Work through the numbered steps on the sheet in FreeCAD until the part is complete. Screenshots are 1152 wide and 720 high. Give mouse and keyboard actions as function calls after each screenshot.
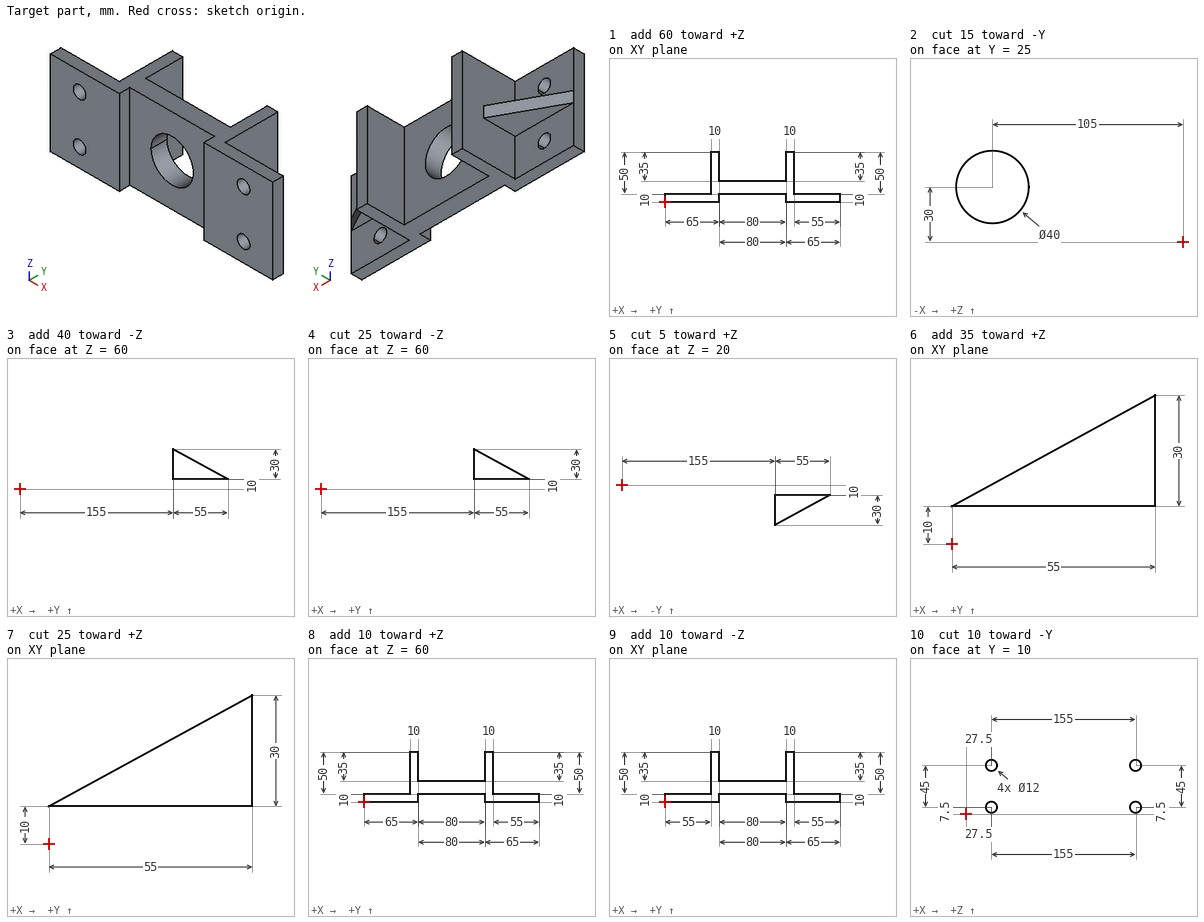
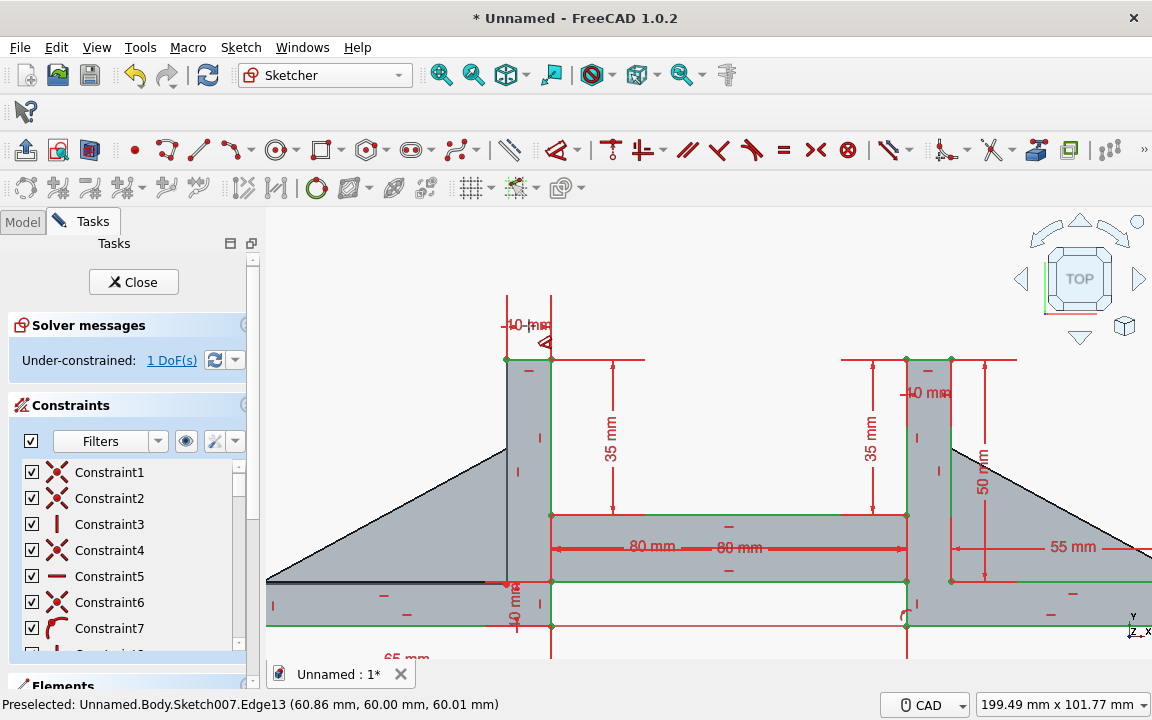
click(507, 427)
click(473, 472)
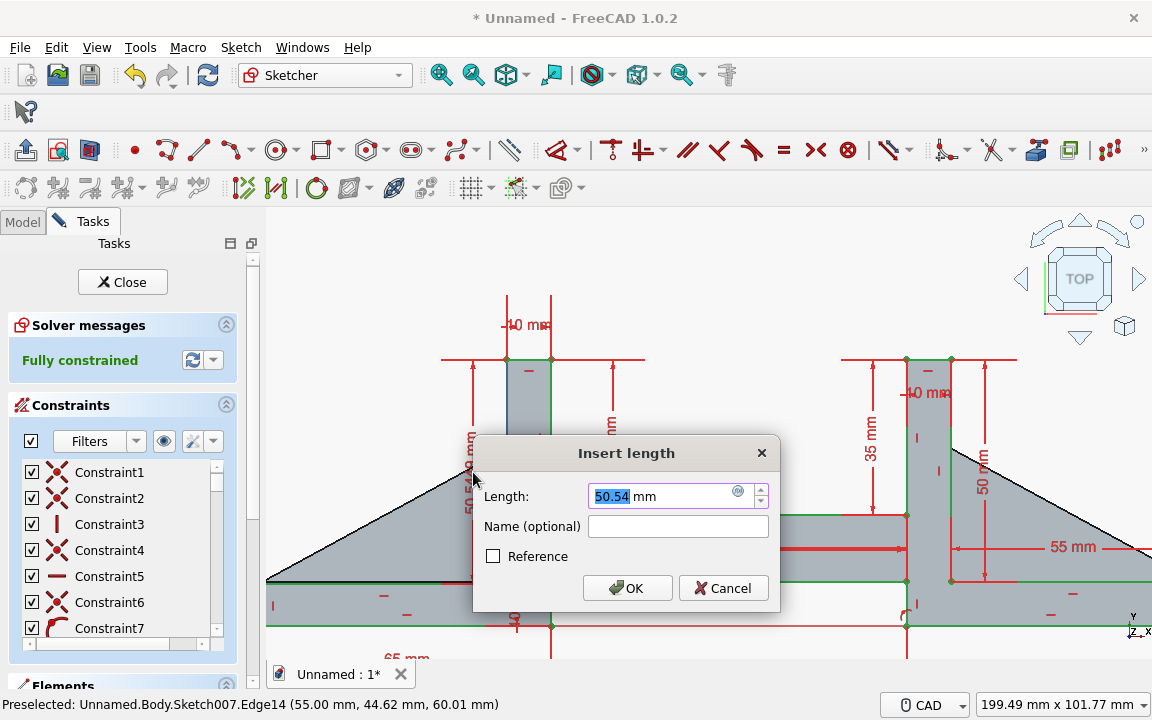
text(50)
key(Return)
key(Escape)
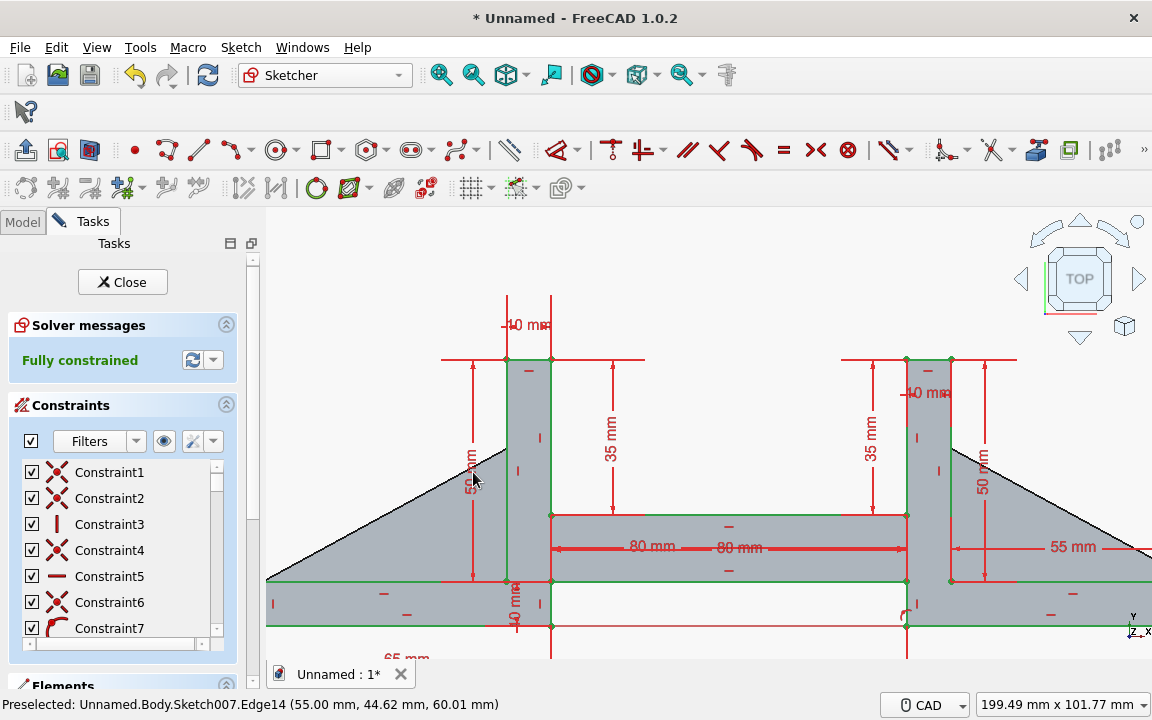
click(123, 282)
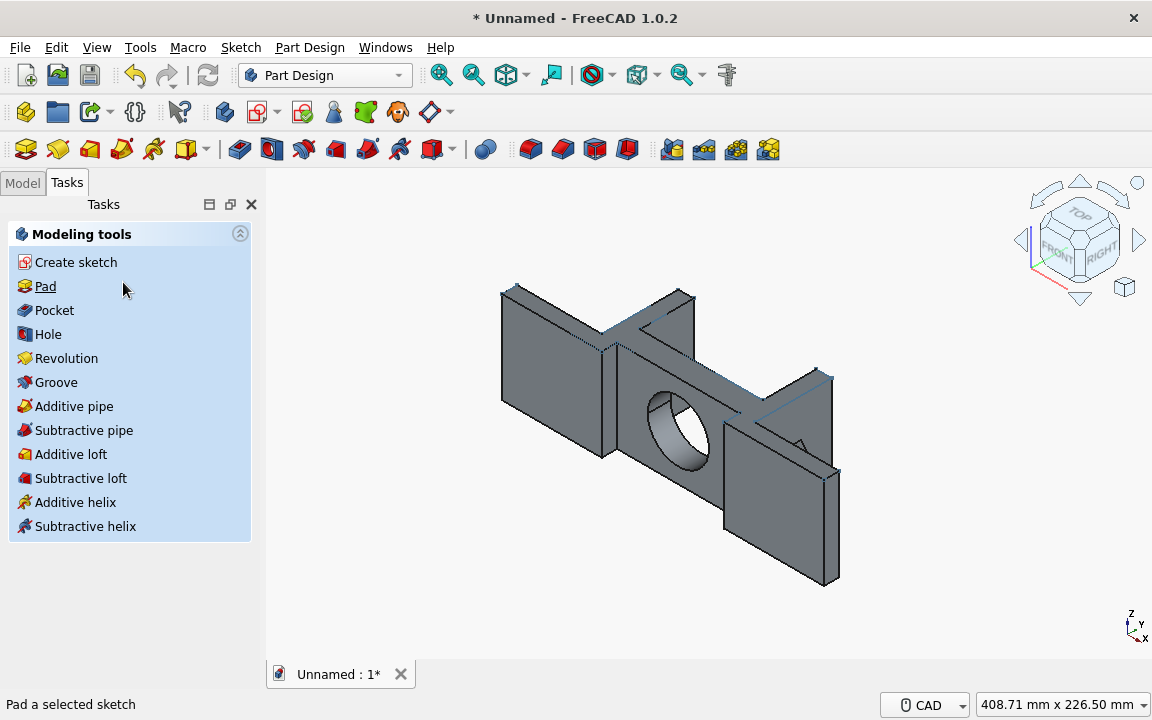
click(26, 150)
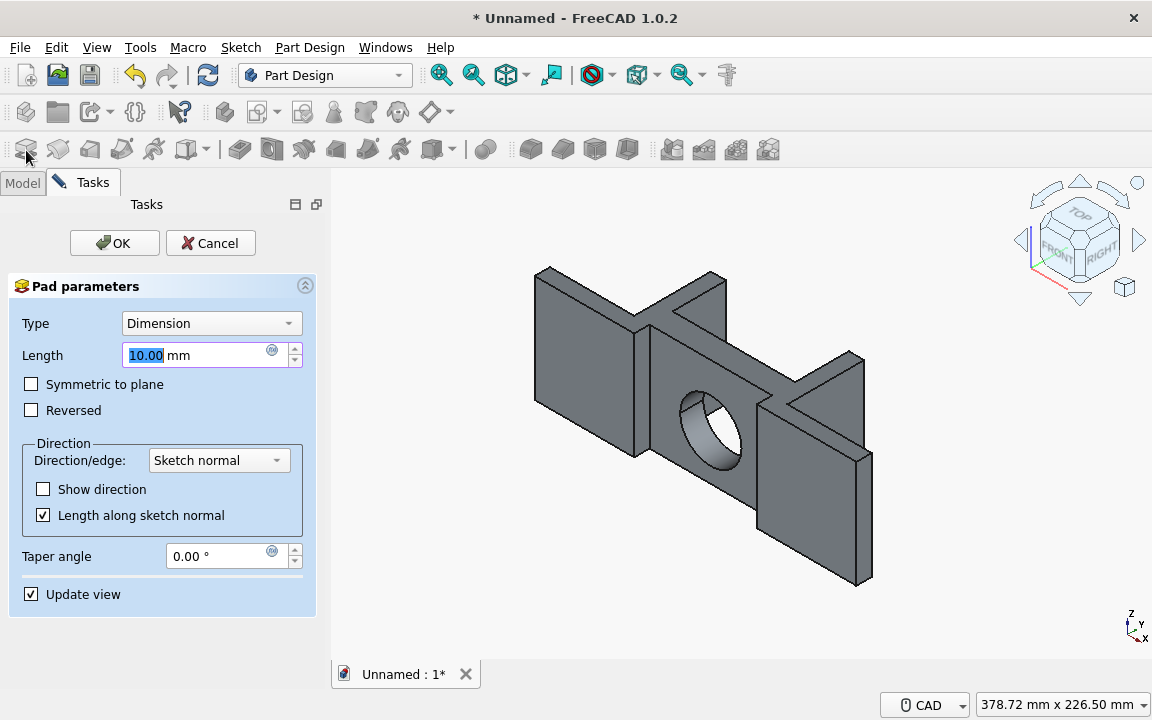
text(10)
key(Tab)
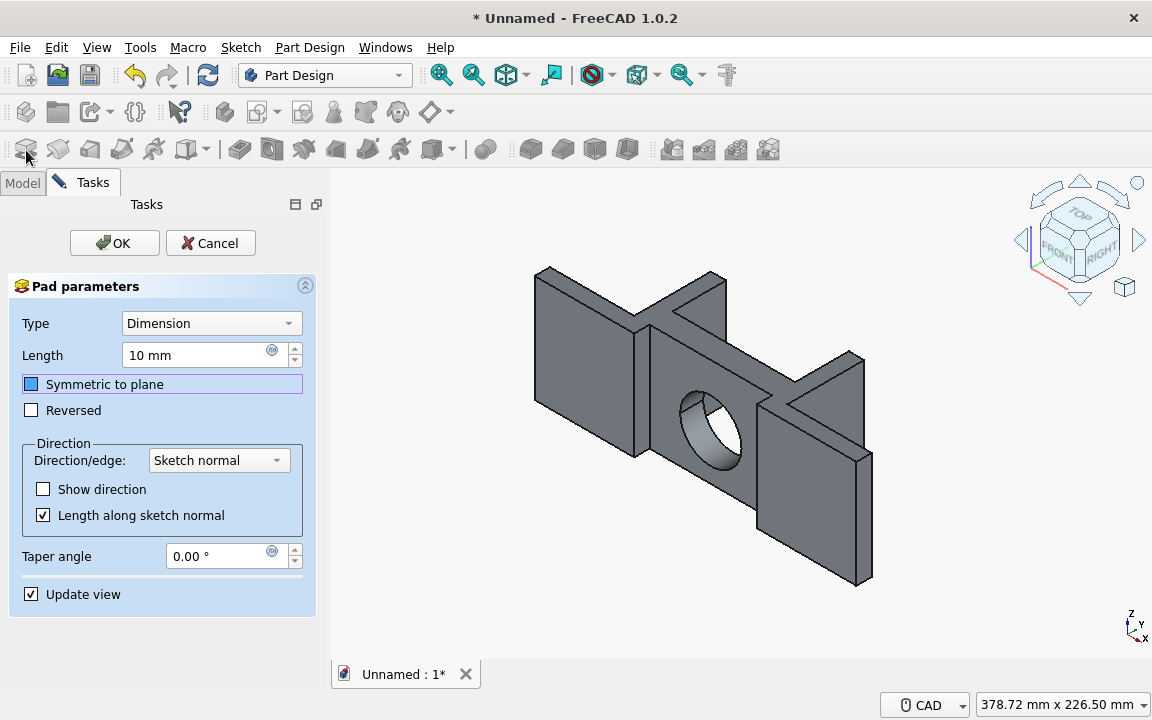
click(115, 243)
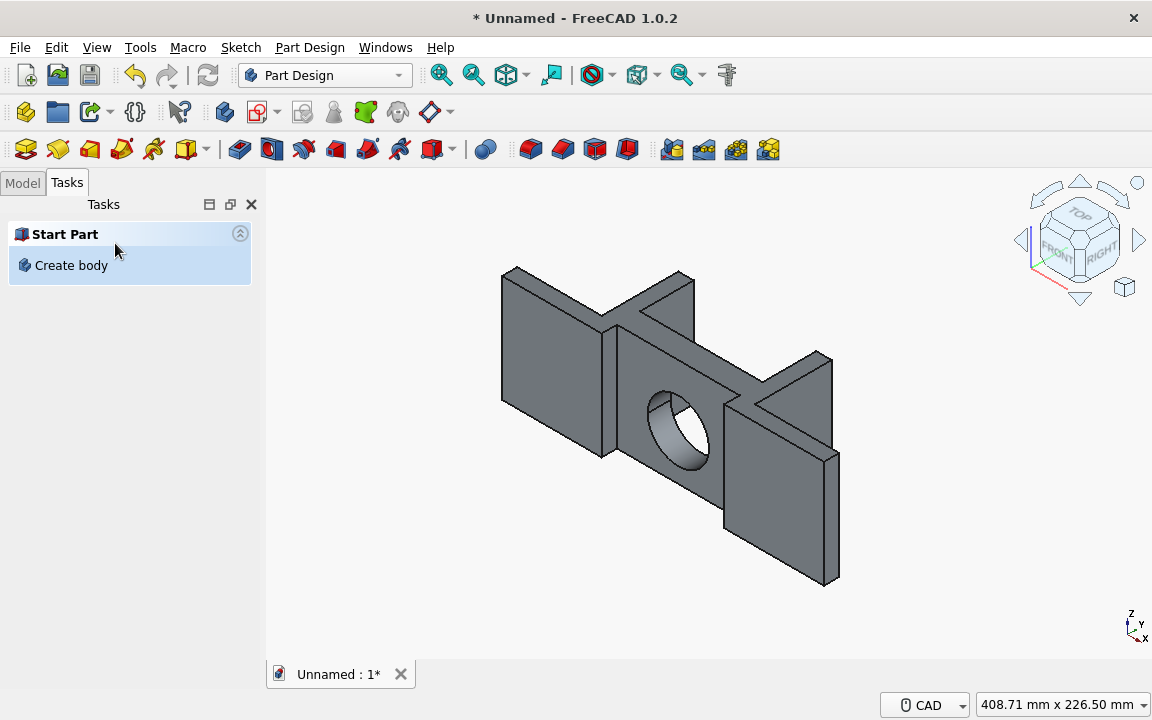
click(258, 112)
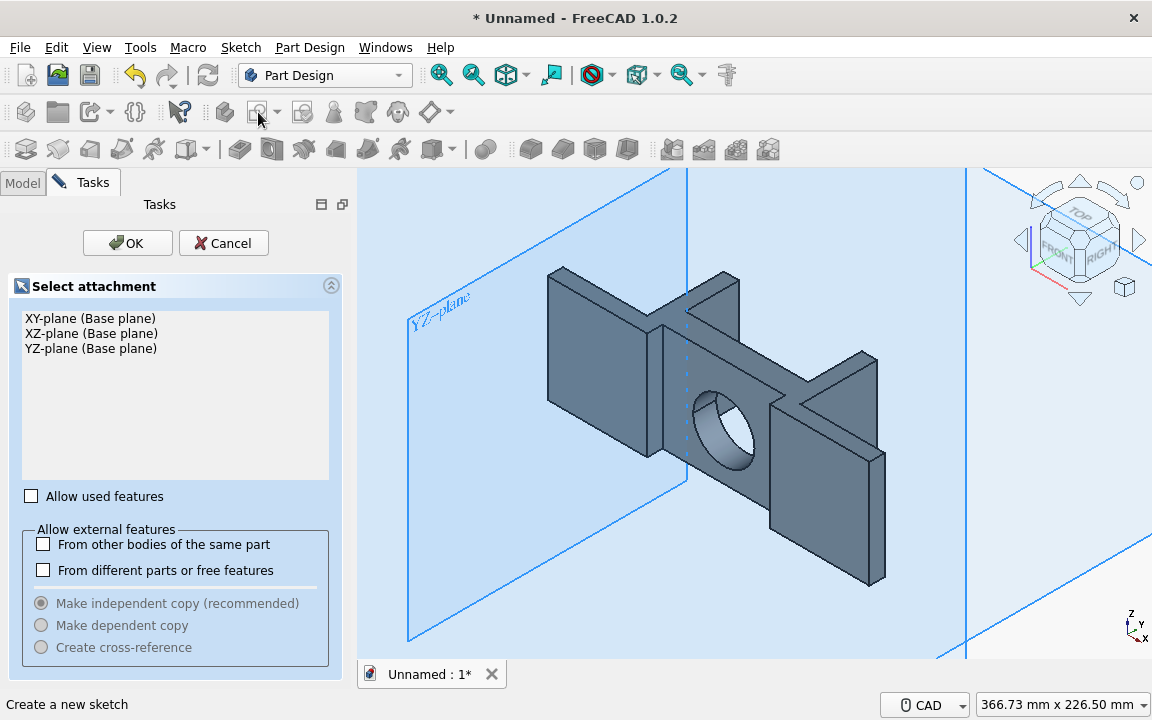
click(82, 318)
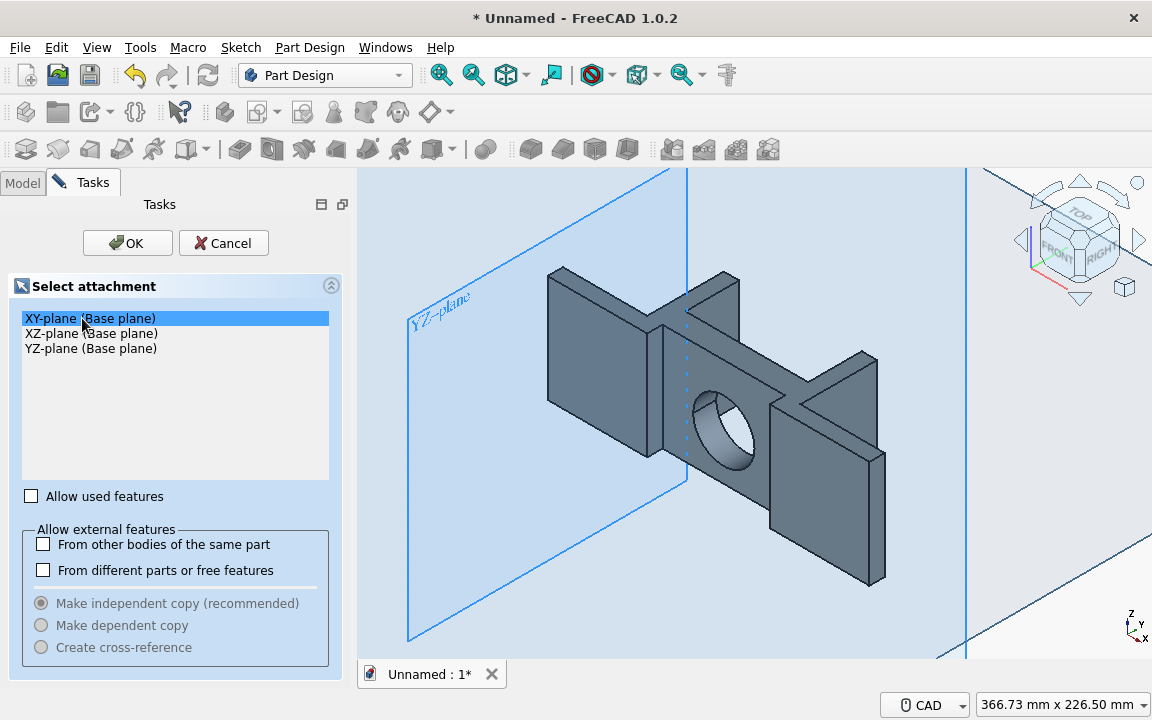
click(128, 243)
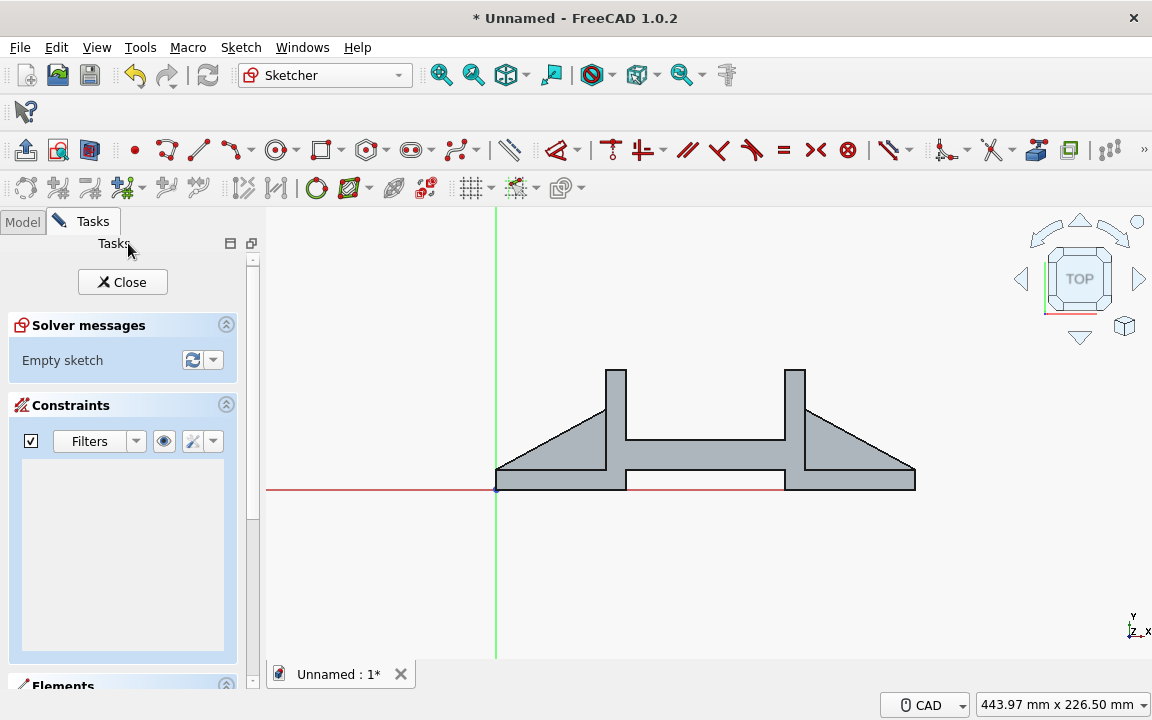
key(q)
key(s)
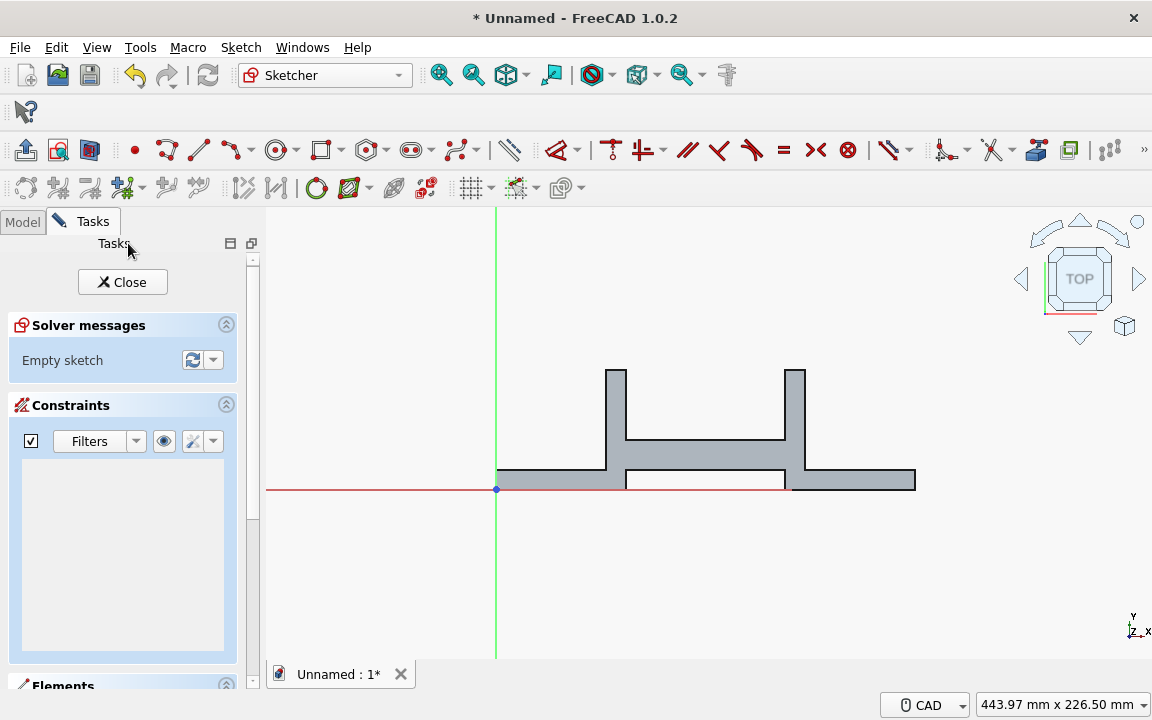
key(g)
key(m)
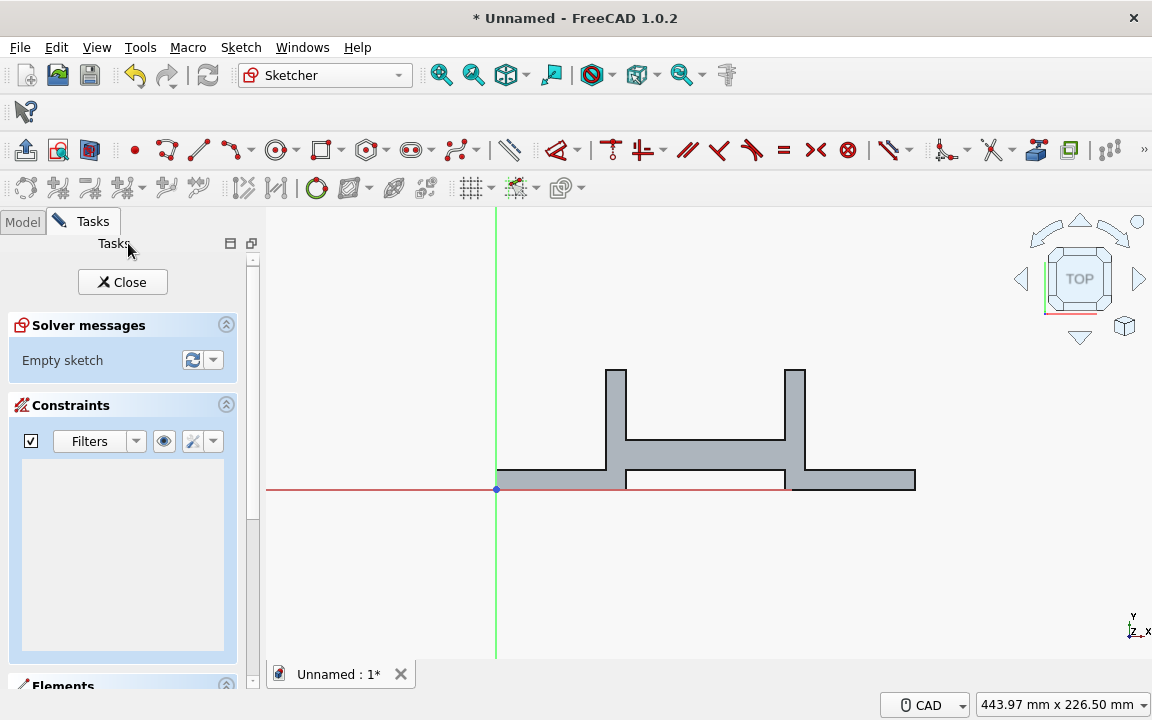
click(496, 490)
click(505, 470)
click(606, 470)
click(606, 370)
click(626, 370)
click(626, 440)
click(785, 440)
click(785, 370)
click(805, 370)
click(805, 470)
click(915, 470)
click(915, 490)
click(785, 481)
click(785, 470)
click(626, 470)
click(626, 481)